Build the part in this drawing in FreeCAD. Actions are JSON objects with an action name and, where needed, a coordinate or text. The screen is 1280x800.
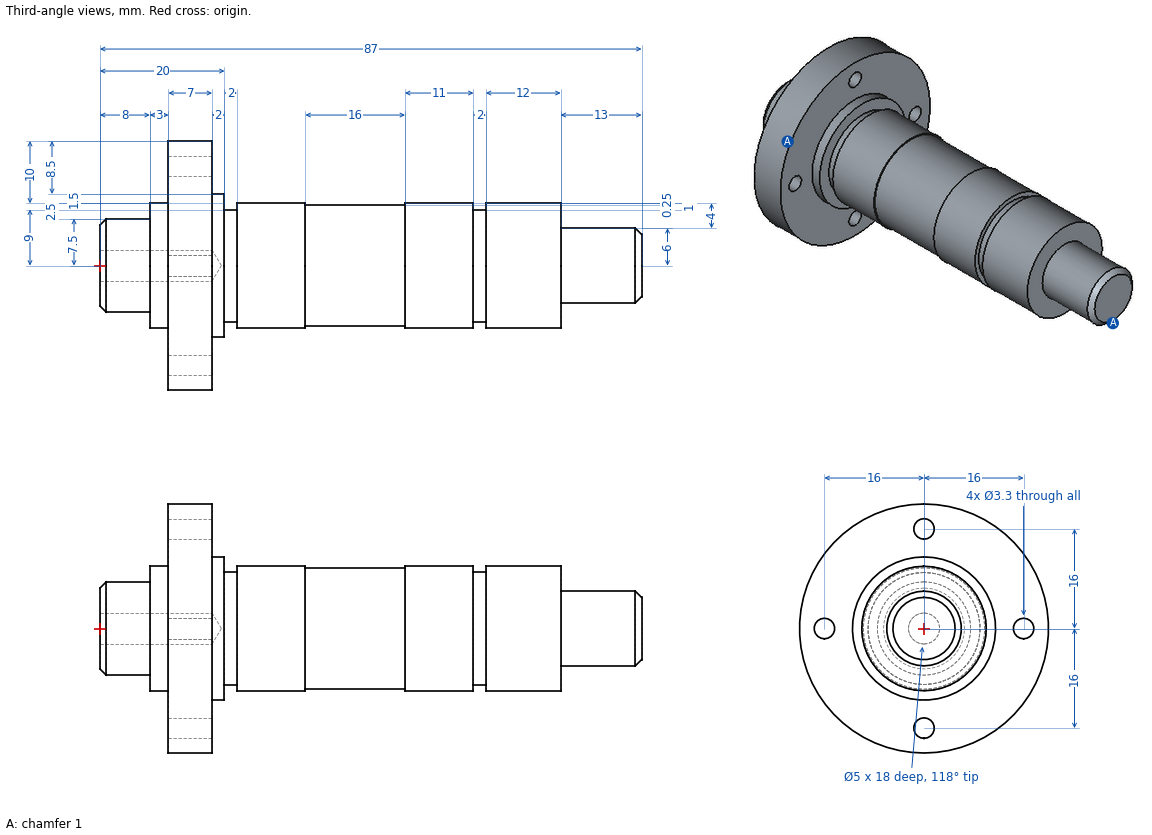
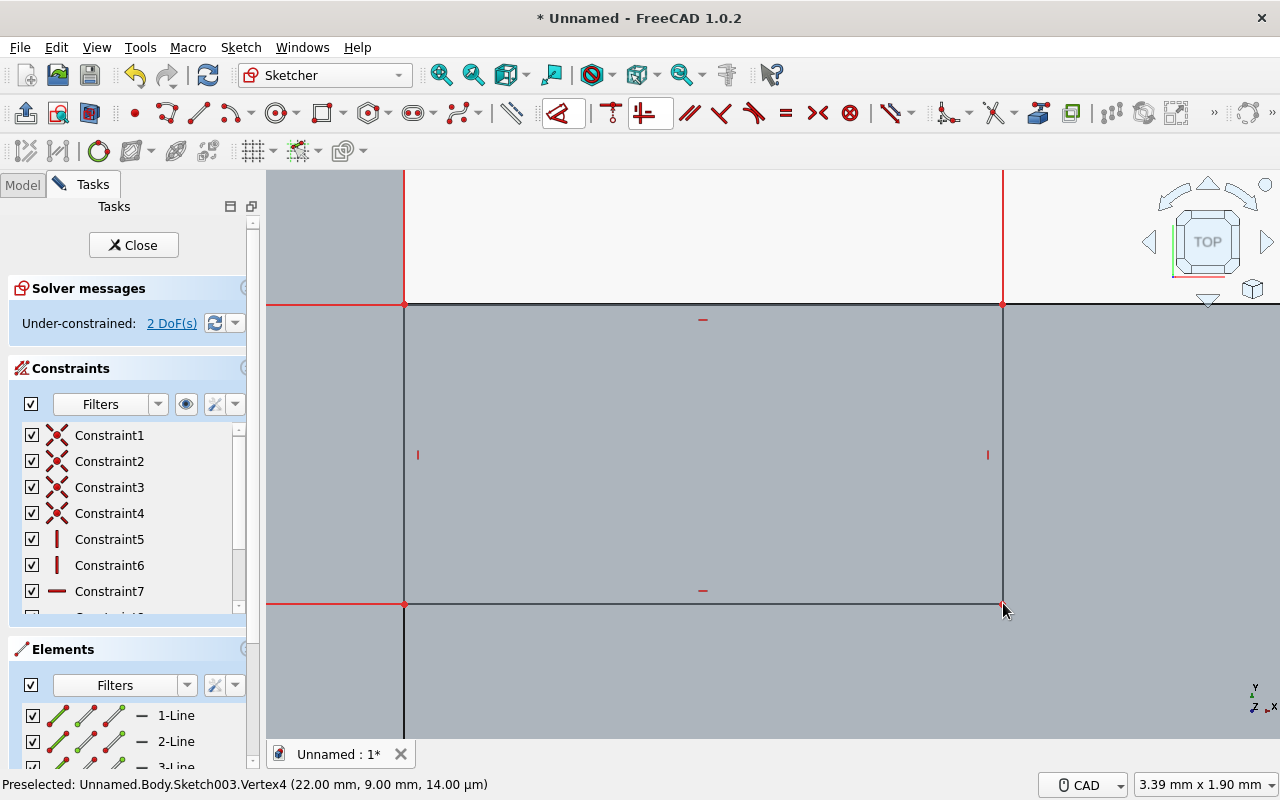
{"action": "left_click", "coordinate": [404, 604]}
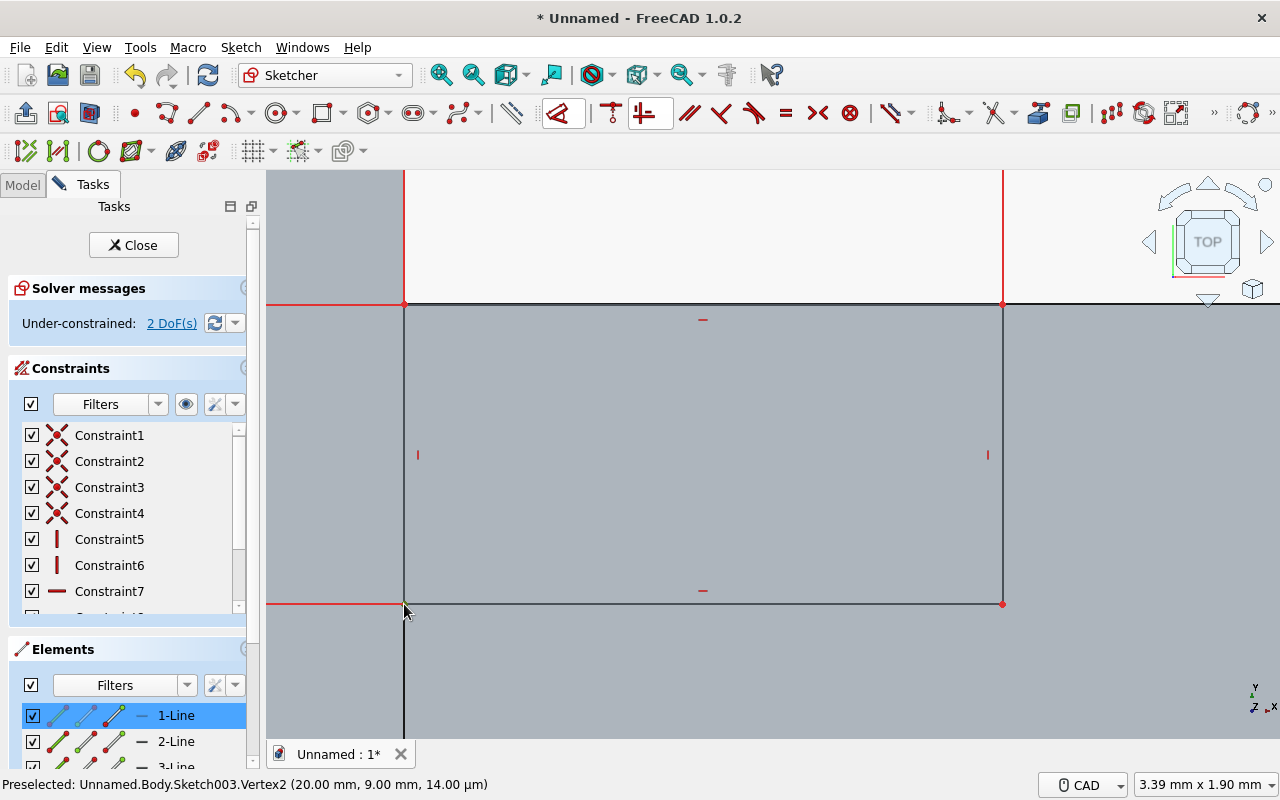
{"action": "key", "text": "i"}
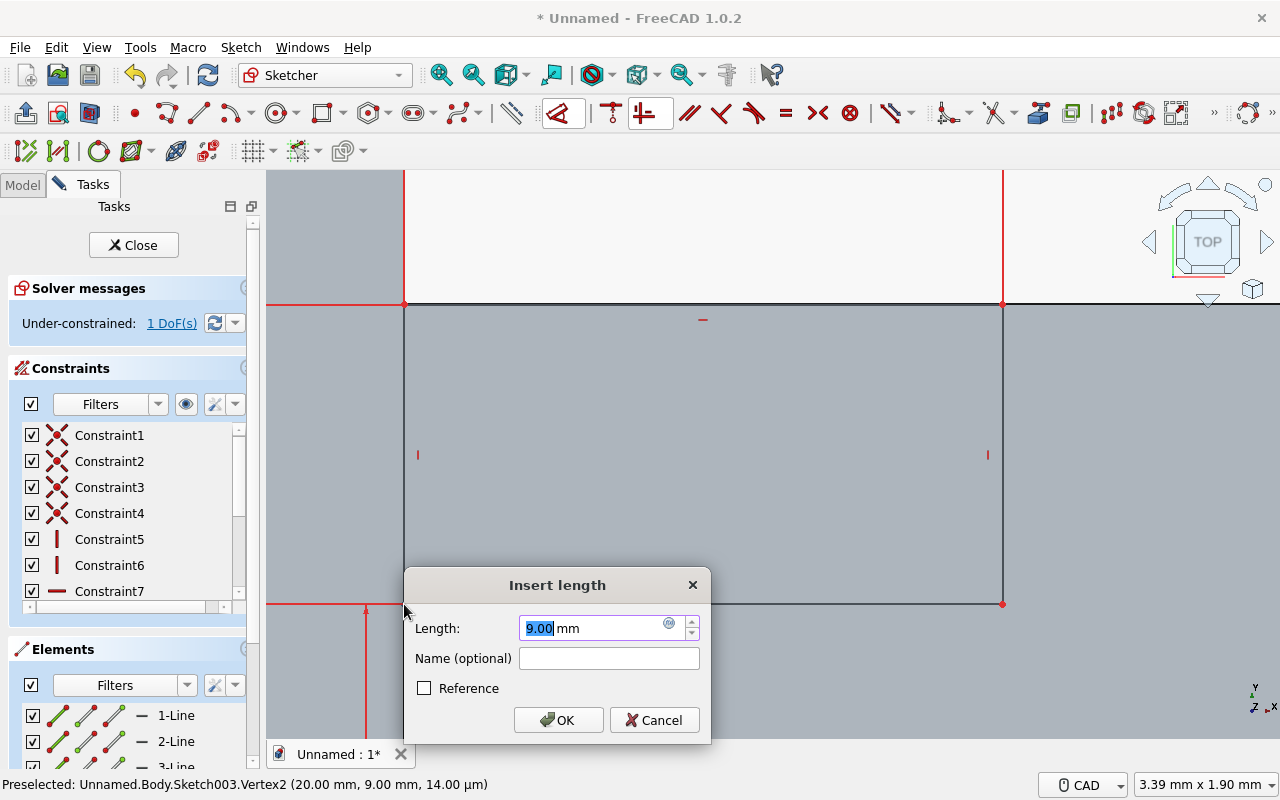
{"action": "type", "text": "9"}
{"action": "key", "text": "Return"}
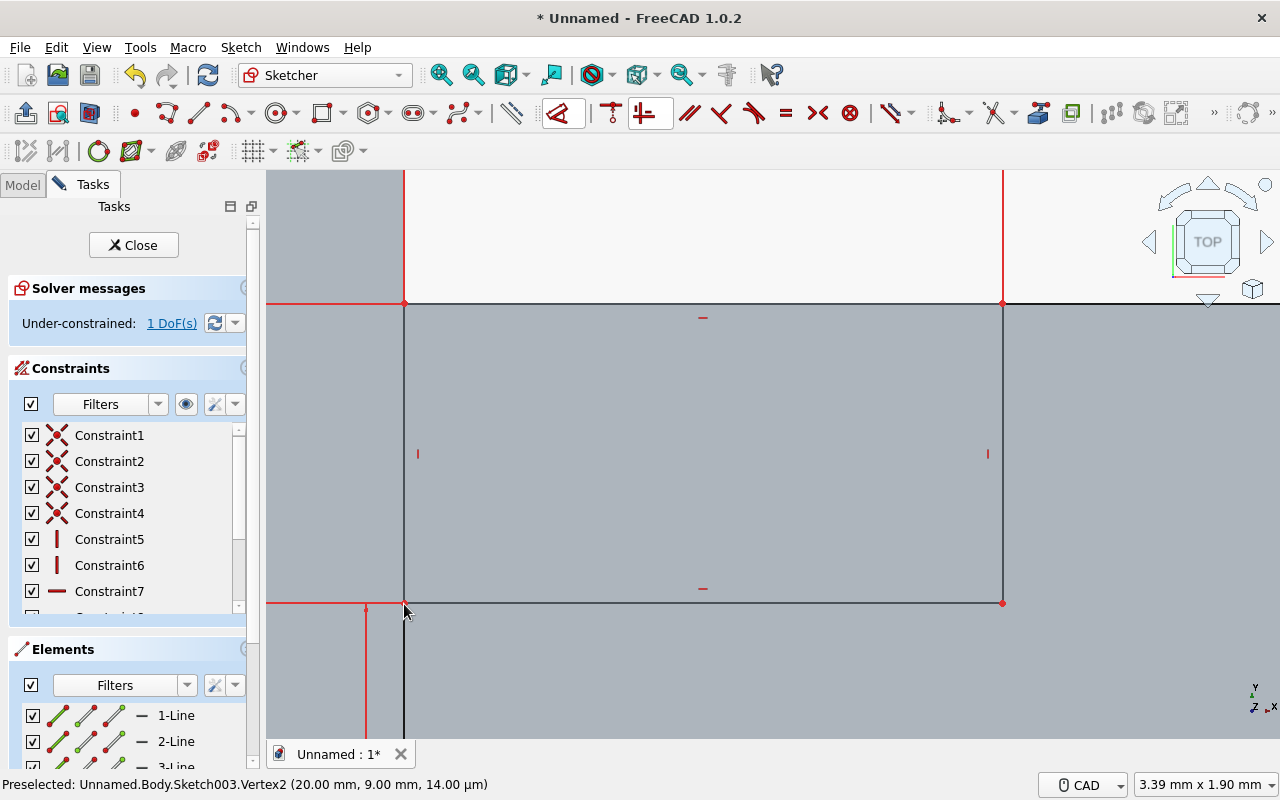
{"action": "left_click", "coordinate": [404, 304]}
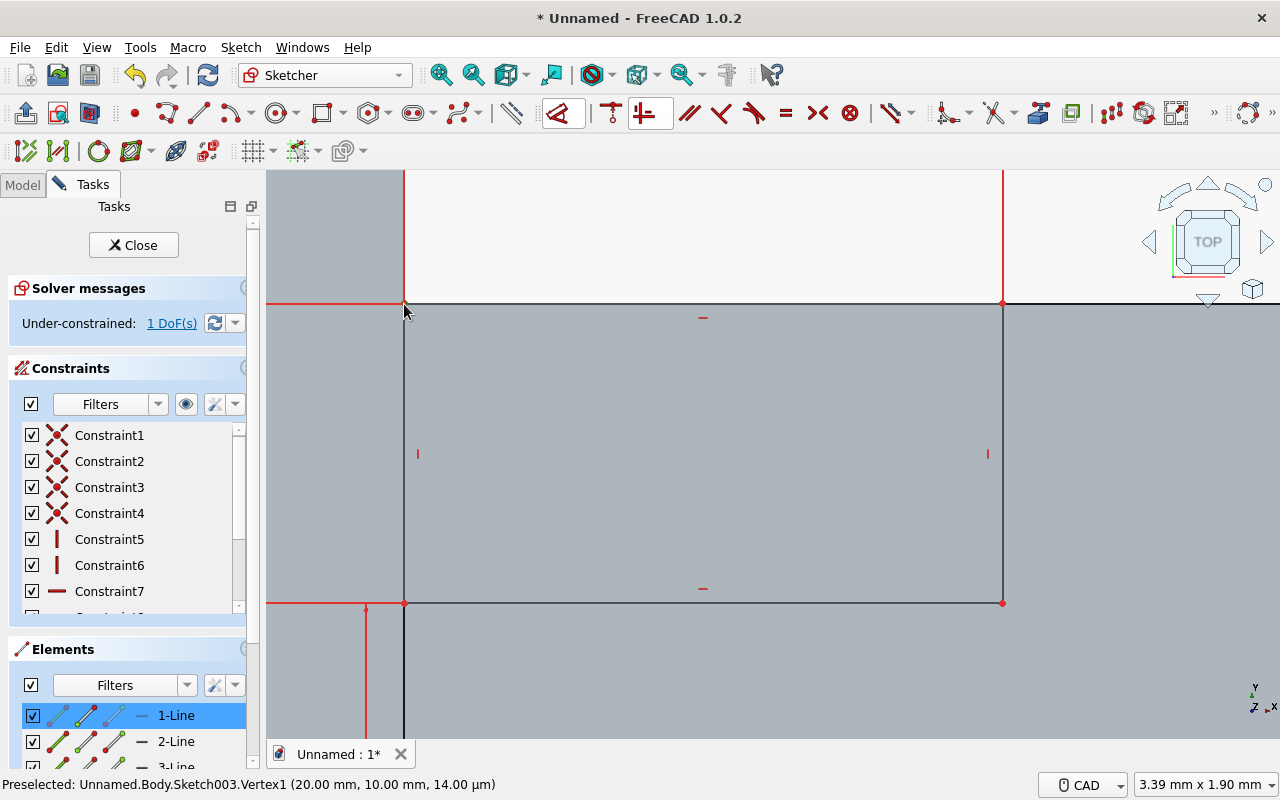
{"action": "left_click", "coordinate": [580, 114]}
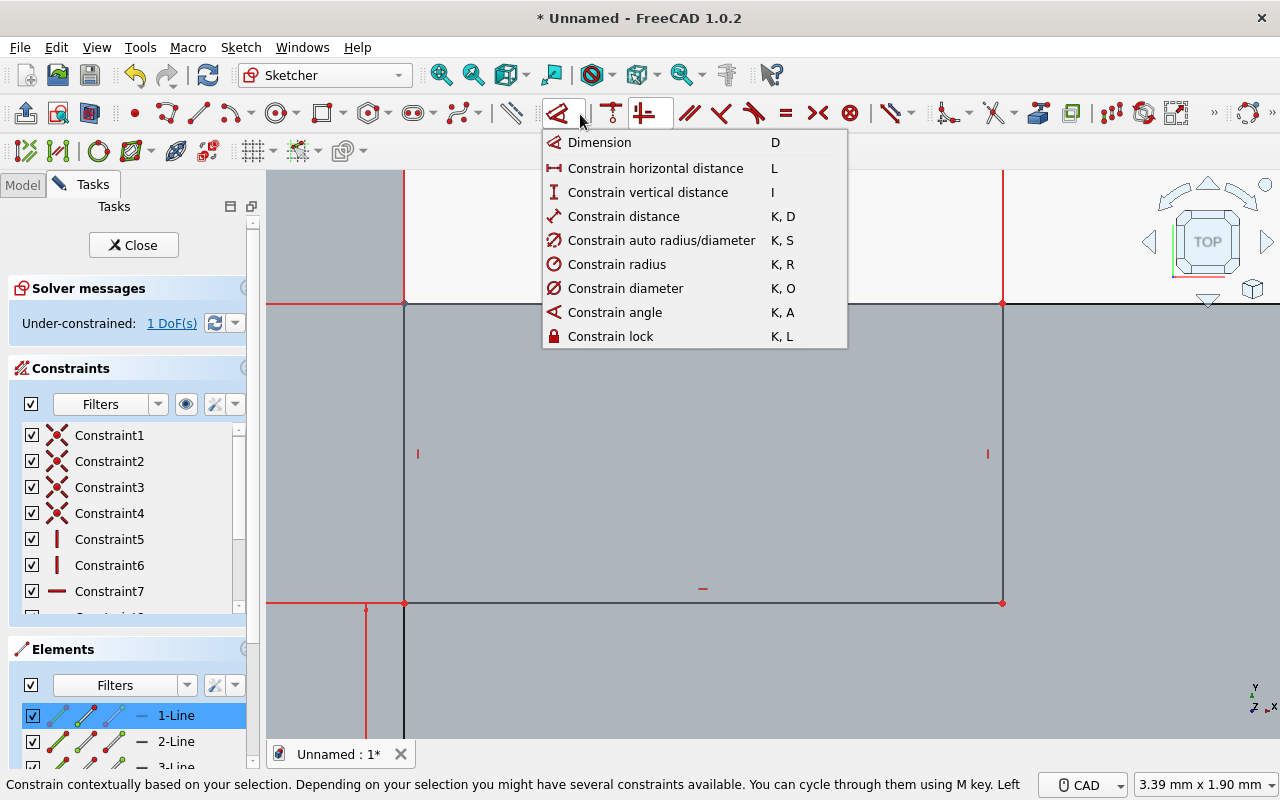
{"action": "left_click", "coordinate": [695, 168]}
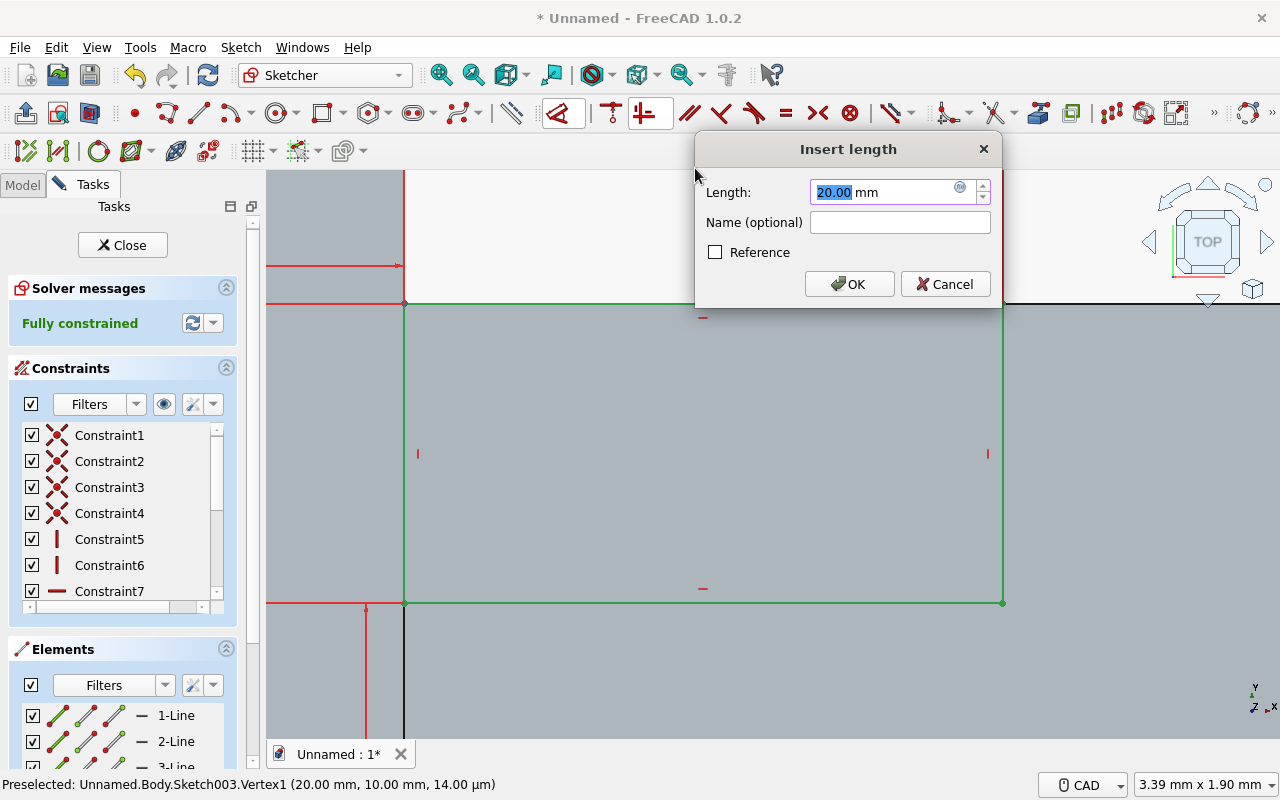
{"action": "type", "text": "20"}
{"action": "key", "text": "Return"}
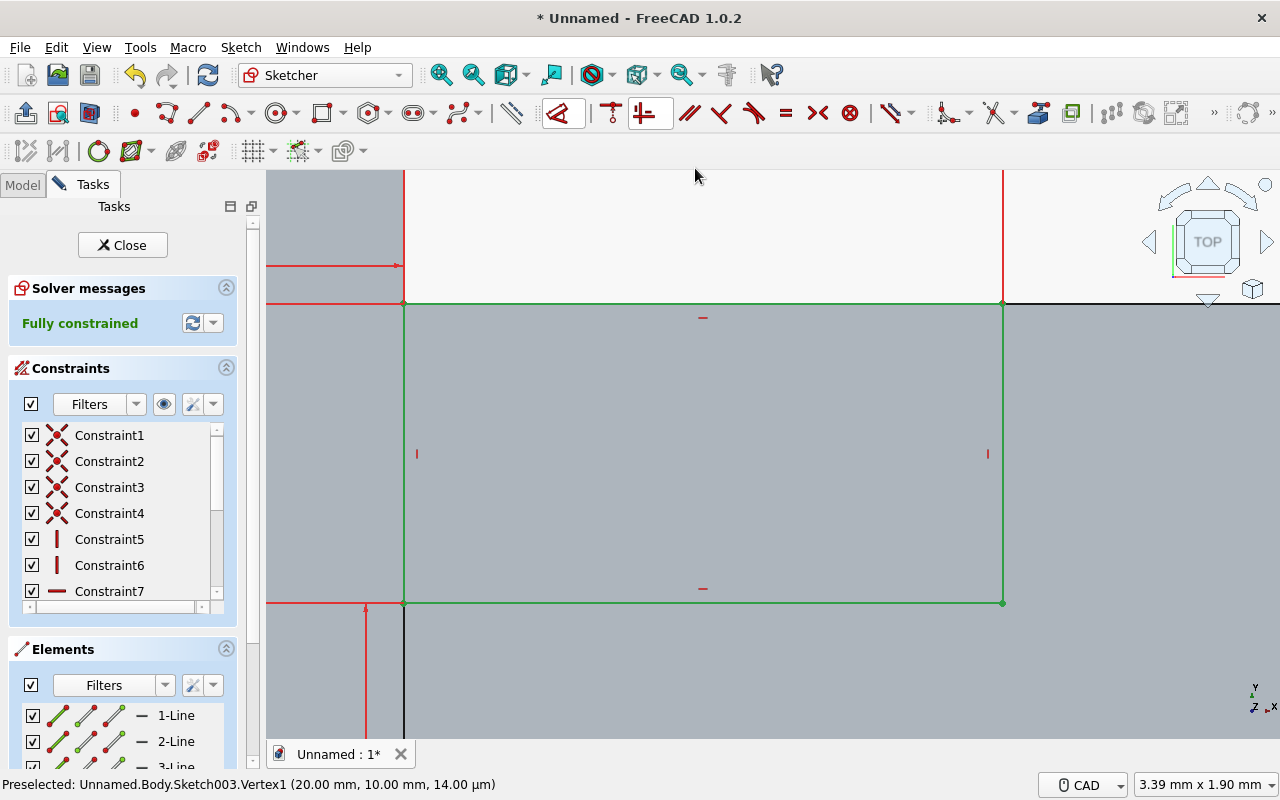
{"action": "left_click", "coordinate": [123, 245]}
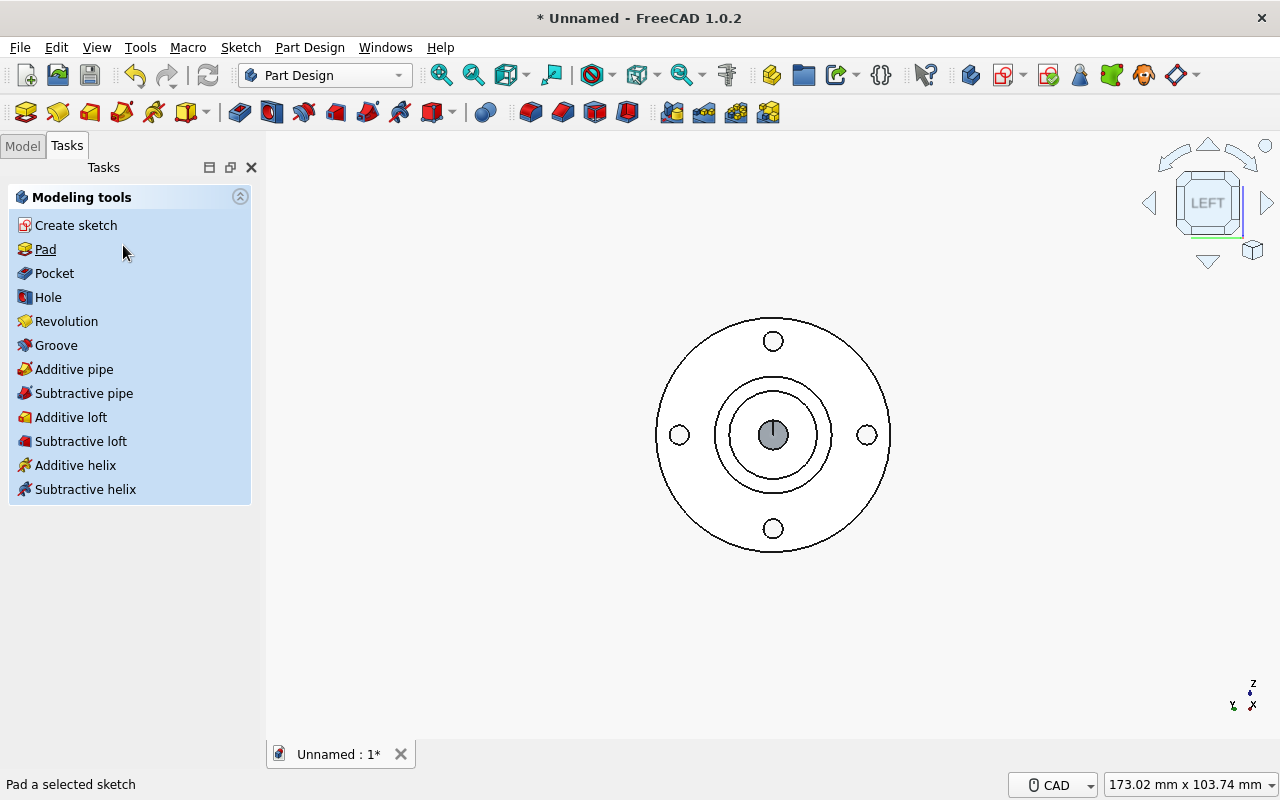
{"action": "left_click", "coordinate": [304, 112]}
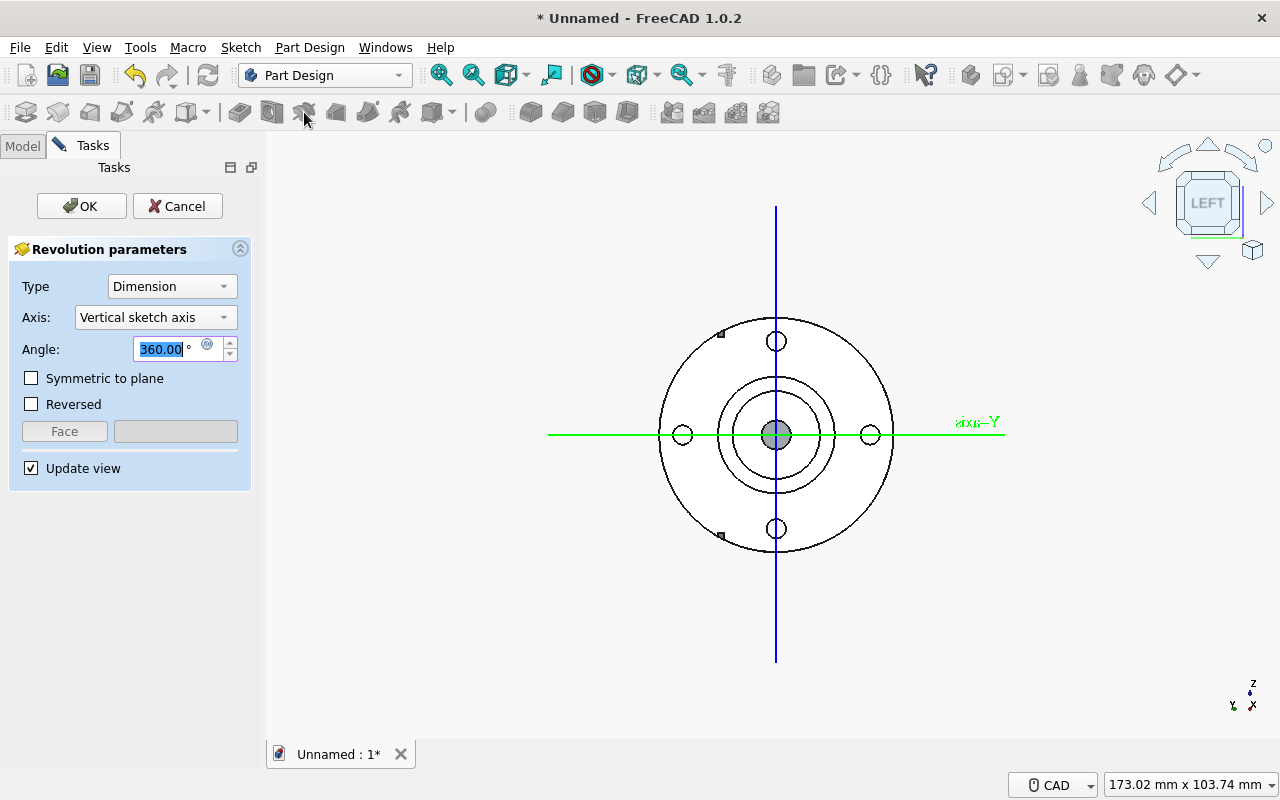
{"action": "left_click", "coordinate": [156, 318]}